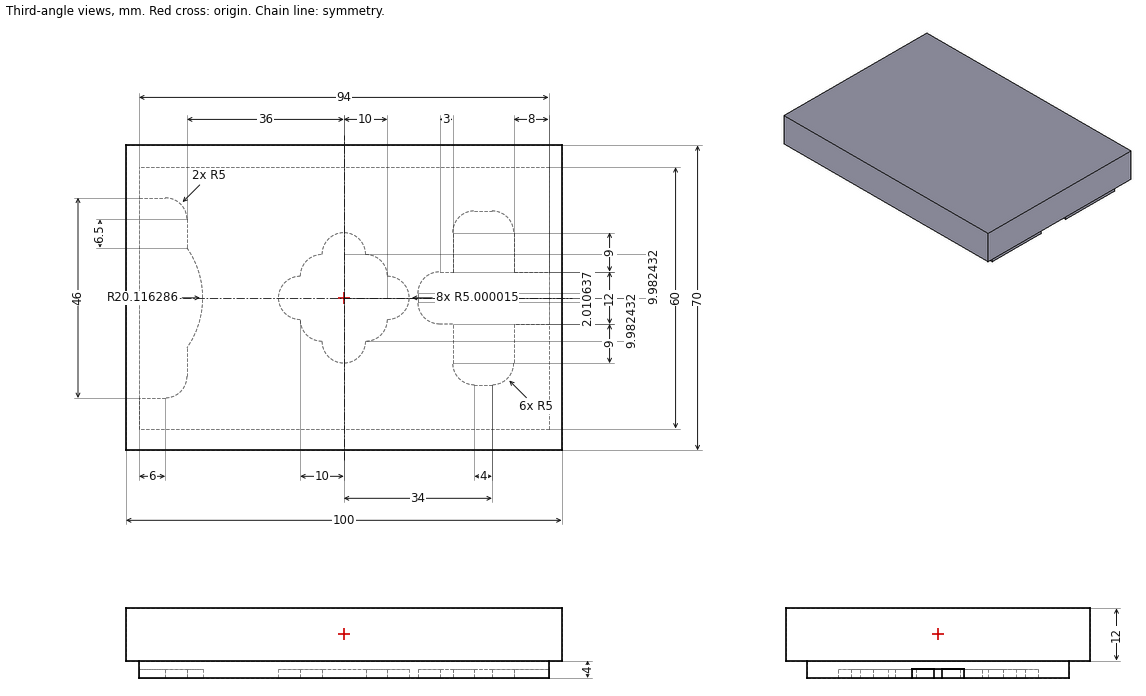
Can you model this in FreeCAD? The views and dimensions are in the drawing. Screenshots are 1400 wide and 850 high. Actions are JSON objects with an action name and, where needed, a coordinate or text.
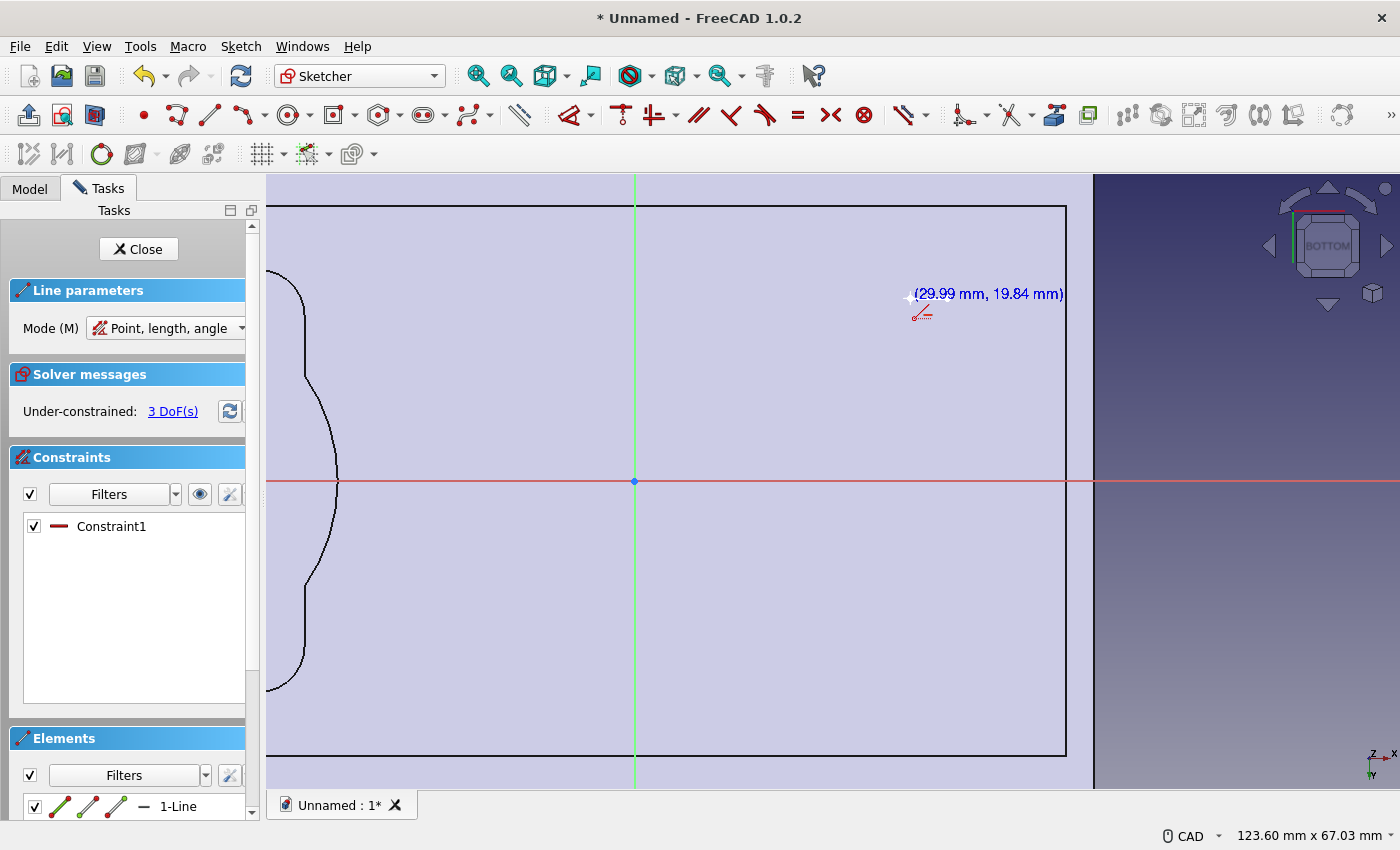
{"action": "left_click", "coordinate": [177, 116]}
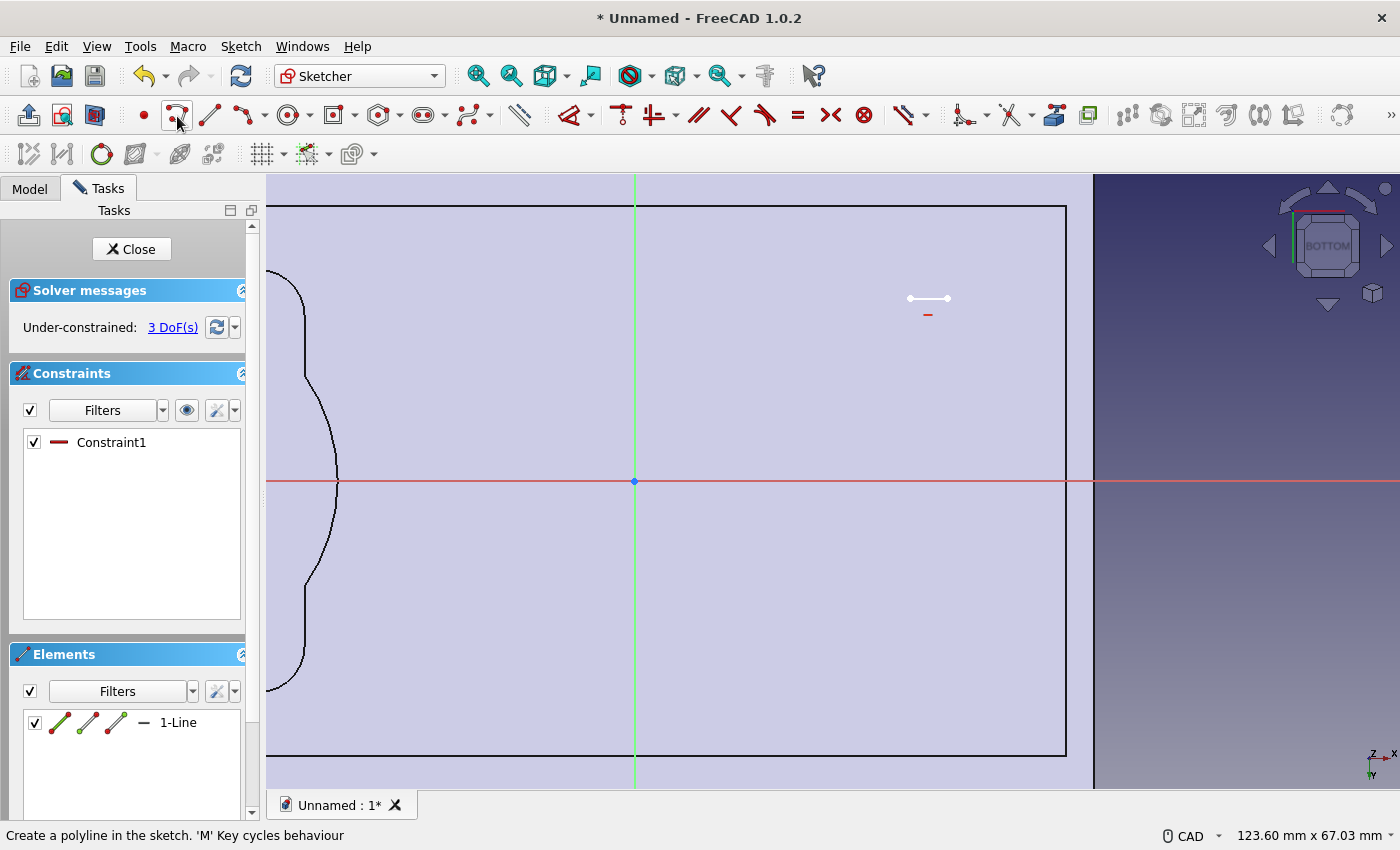
{"action": "left_click", "coordinate": [864, 343]}
{"action": "left_click", "coordinate": [864, 426]}
{"action": "left_click", "coordinate": [837, 423]}
{"action": "right_click", "coordinate": [837, 423]}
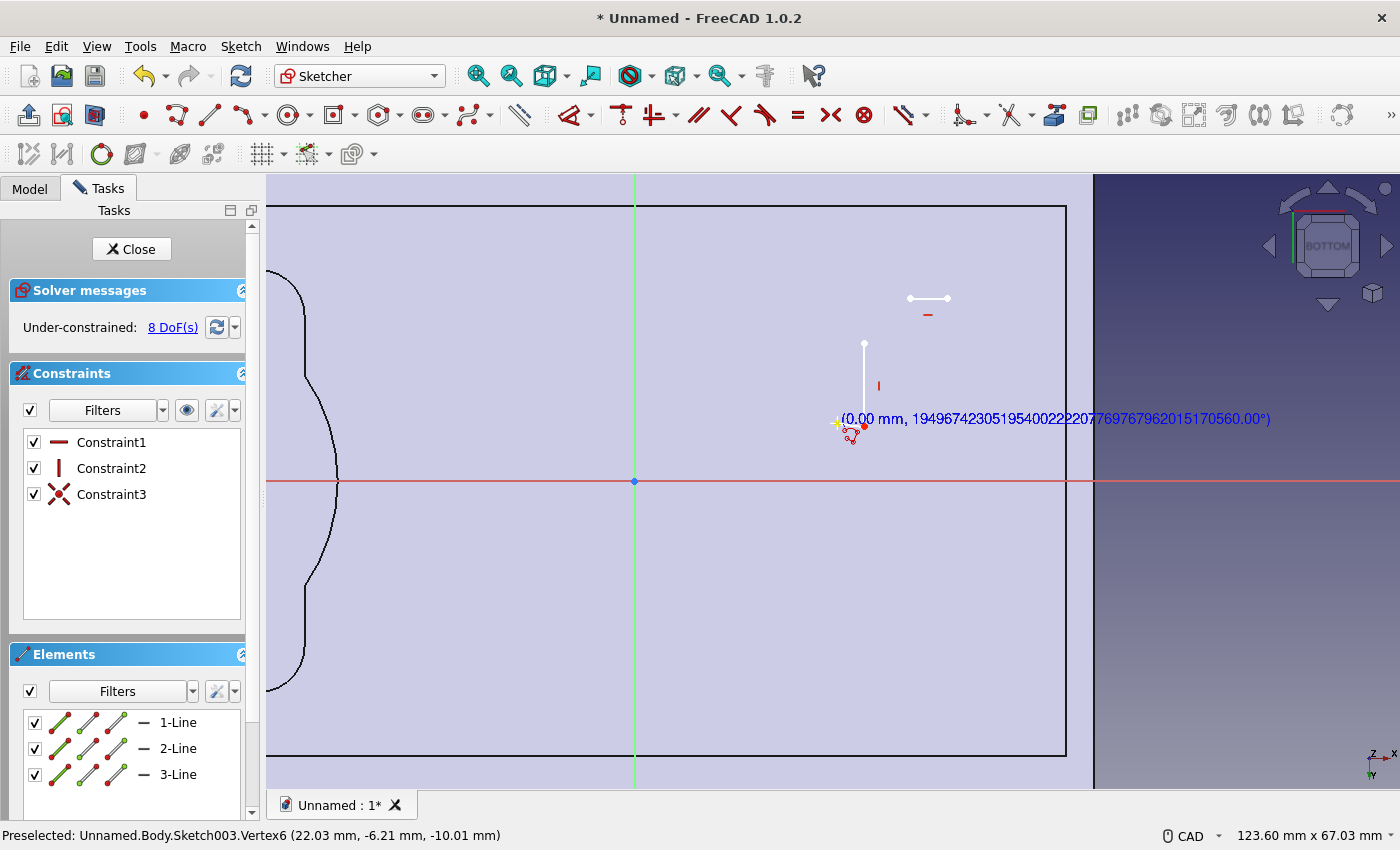
{"action": "left_click", "coordinate": [210, 116]}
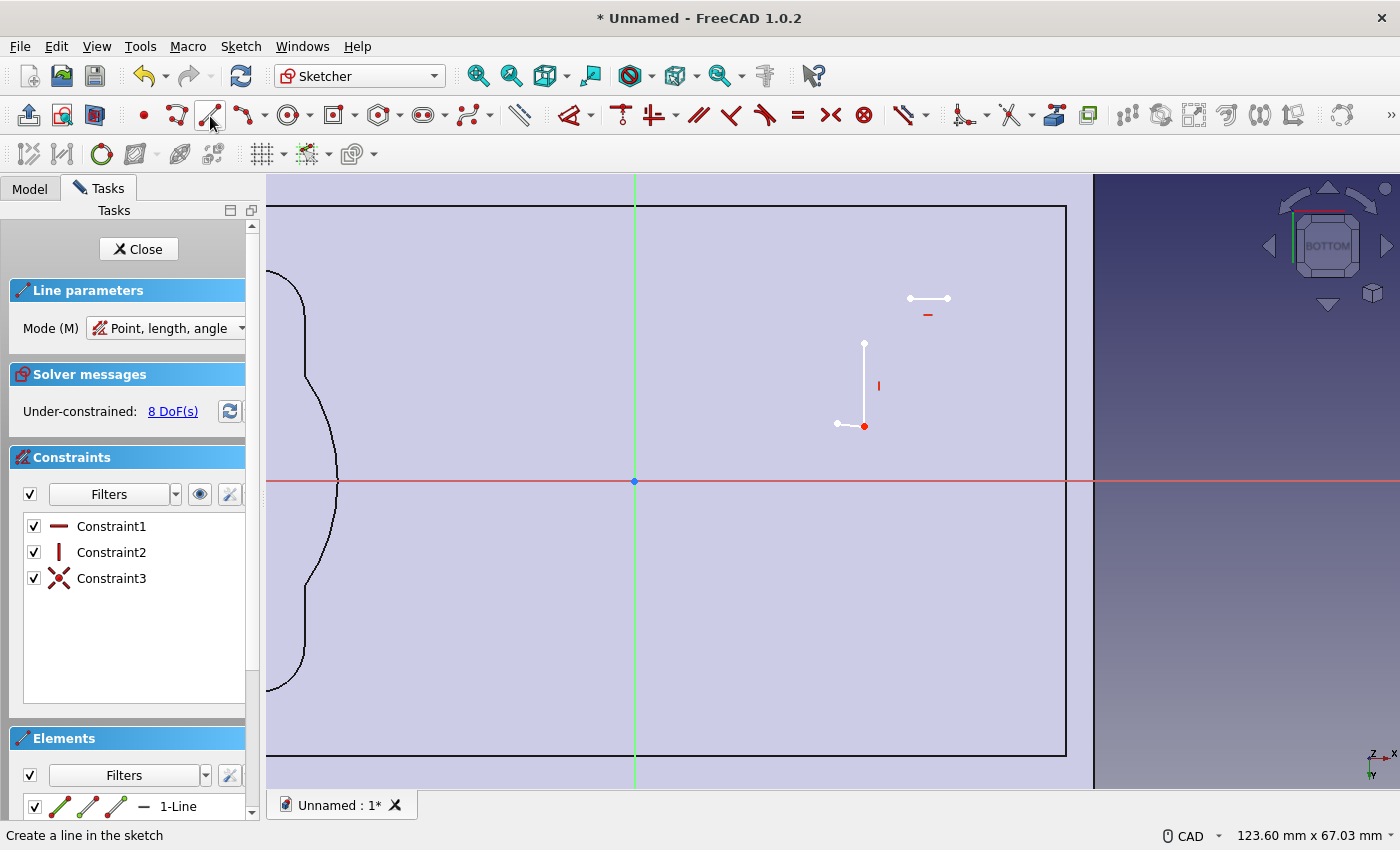
{"action": "scroll", "coordinate": [791, 472], "scroll_direction": "up", "scroll_amount": 3}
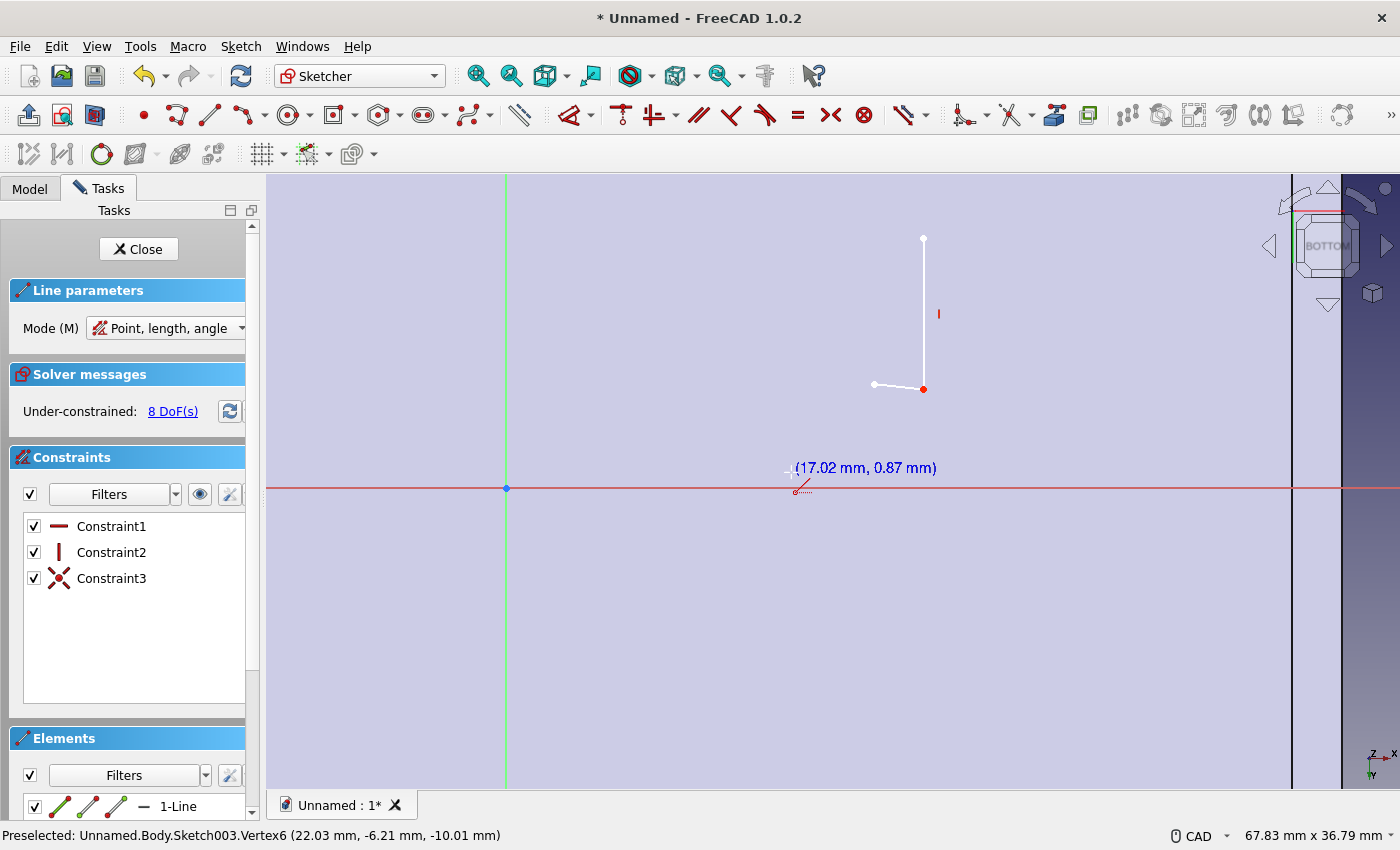
{"action": "left_click", "coordinate": [790, 471]}
{"action": "left_click", "coordinate": [790, 505]}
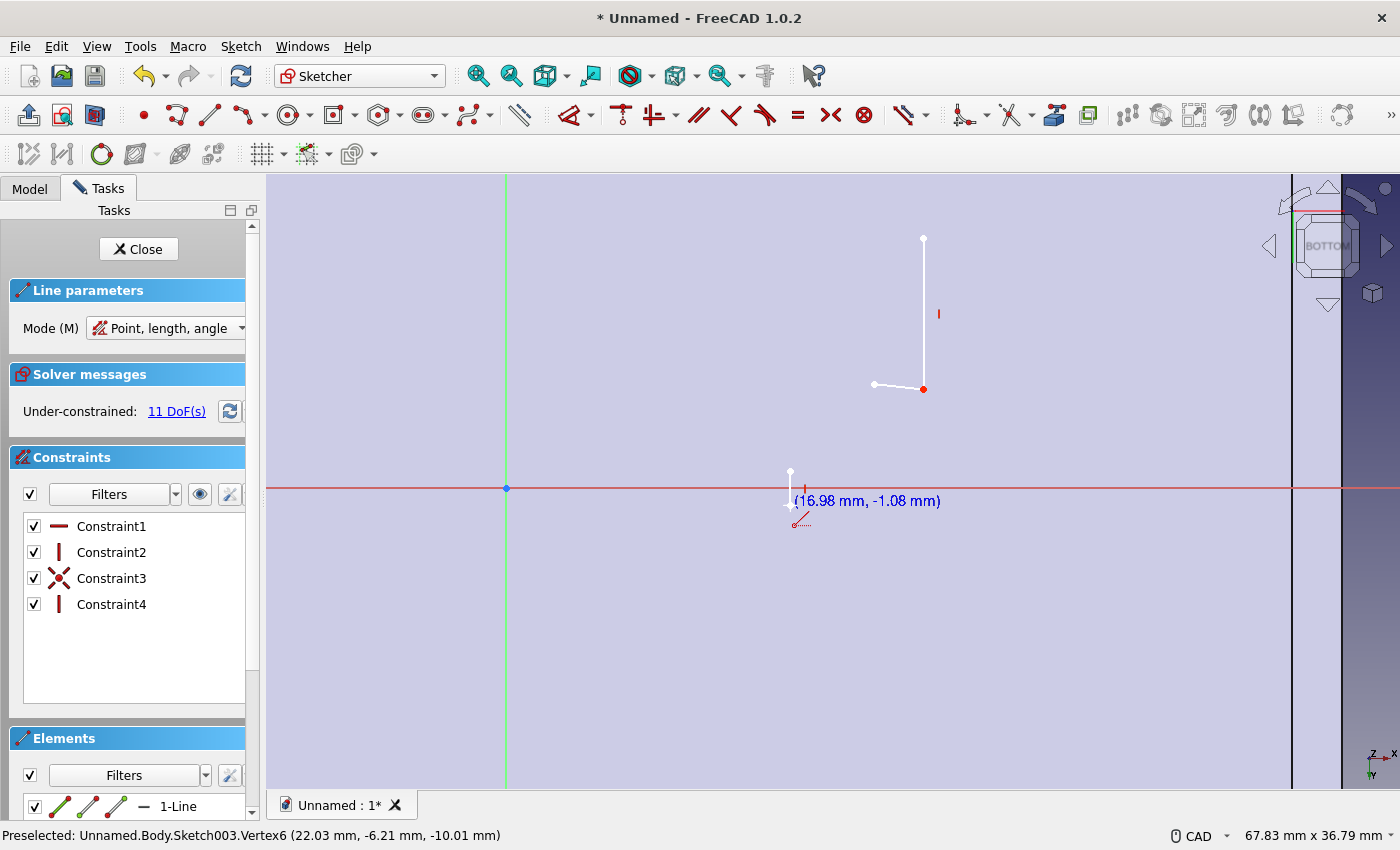
{"action": "left_click", "coordinate": [177, 116]}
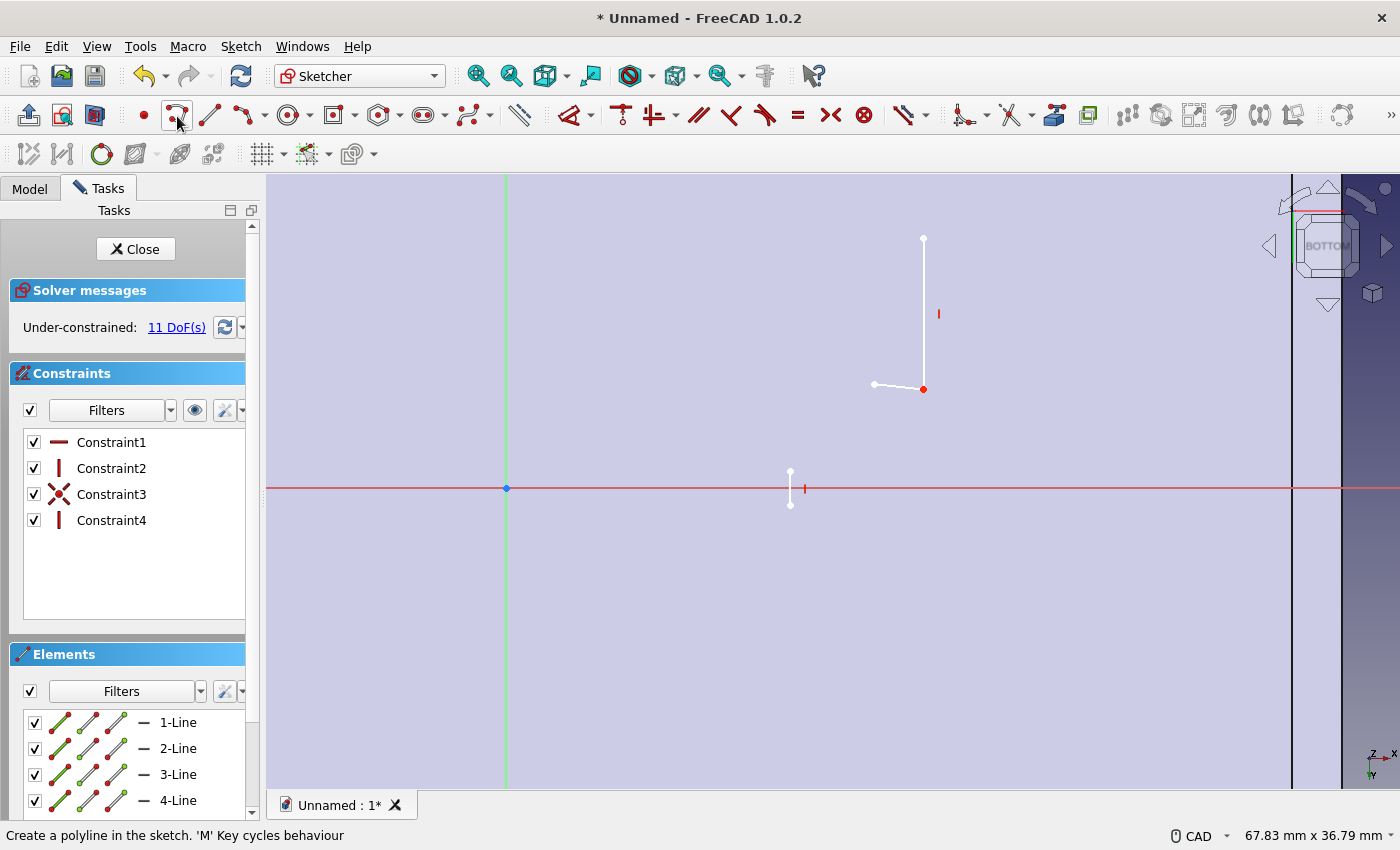
{"action": "left_click", "coordinate": [874, 588]}
{"action": "left_click", "coordinate": [924, 588]}
{"action": "left_click", "coordinate": [924, 739]}
{"action": "right_click", "coordinate": [924, 739]}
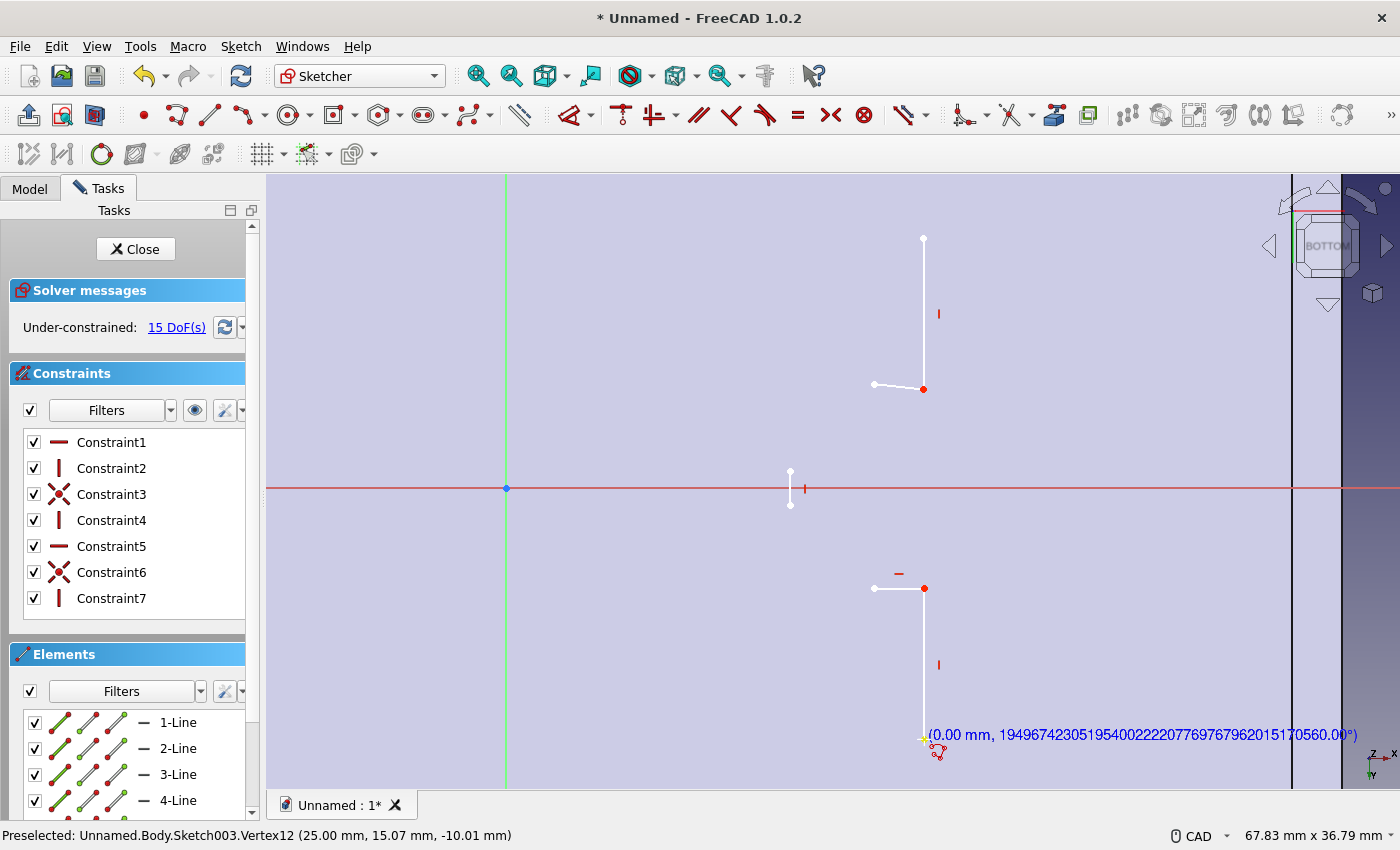
{"action": "left_click", "coordinate": [210, 116]}